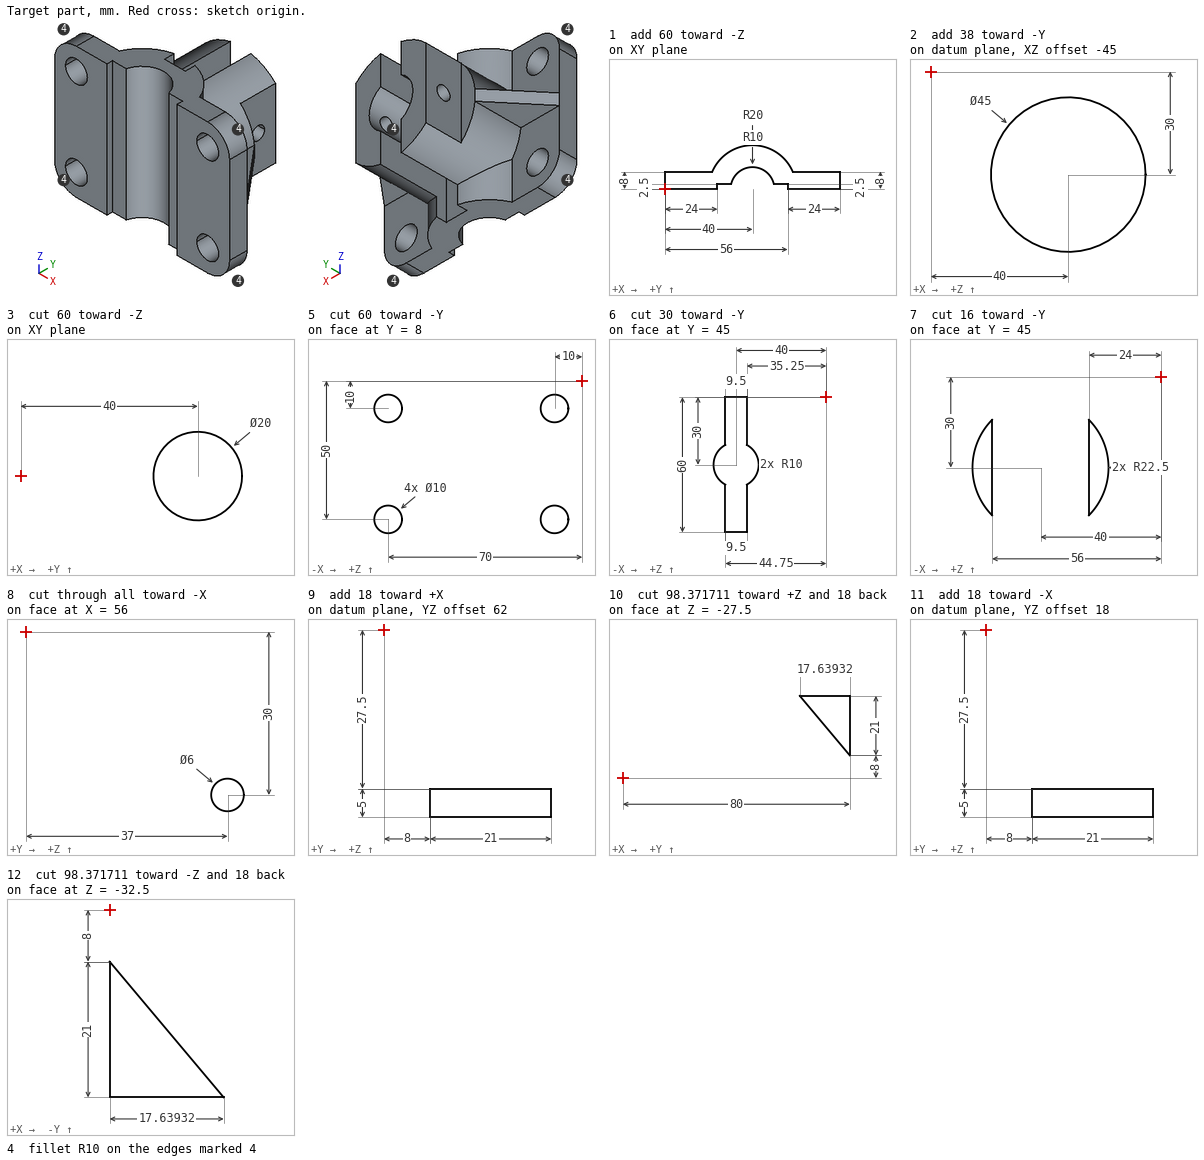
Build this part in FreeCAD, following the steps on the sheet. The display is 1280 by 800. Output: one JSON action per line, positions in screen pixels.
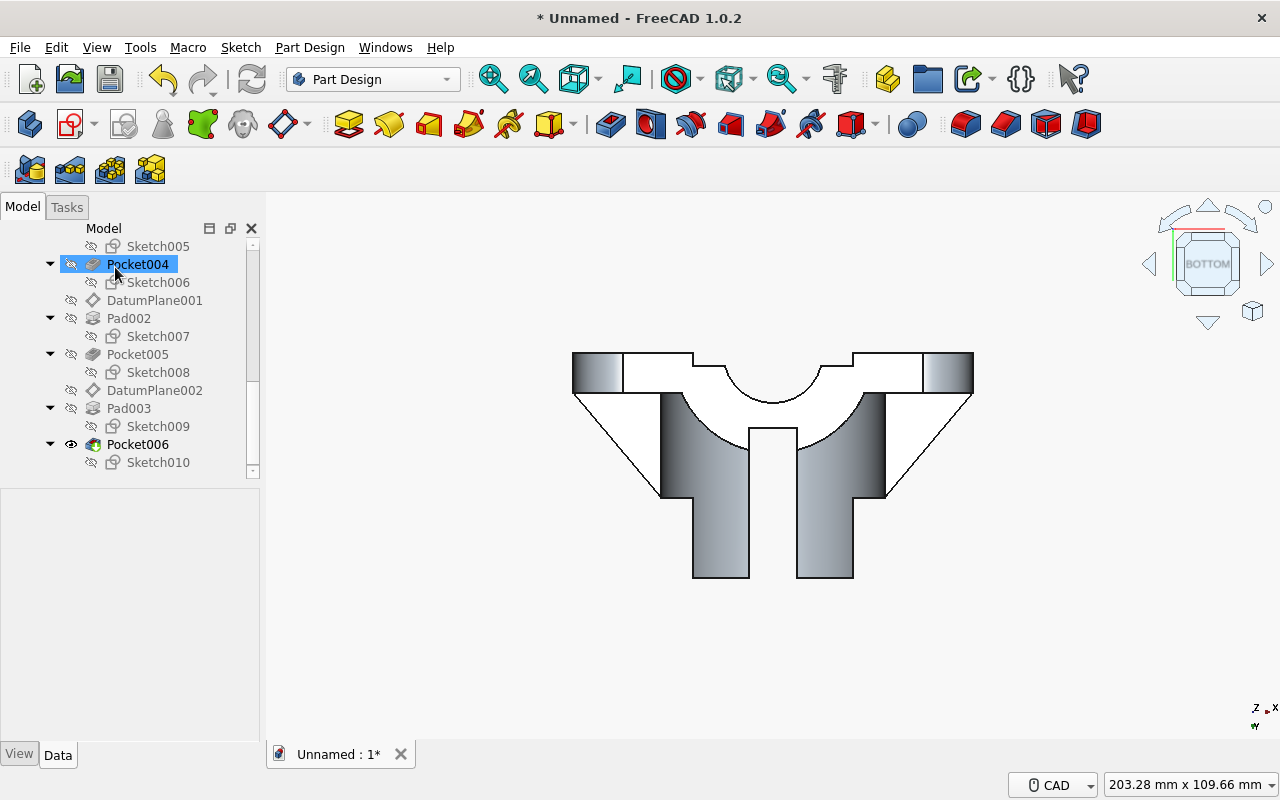
{"action": "key", "text": "0"}